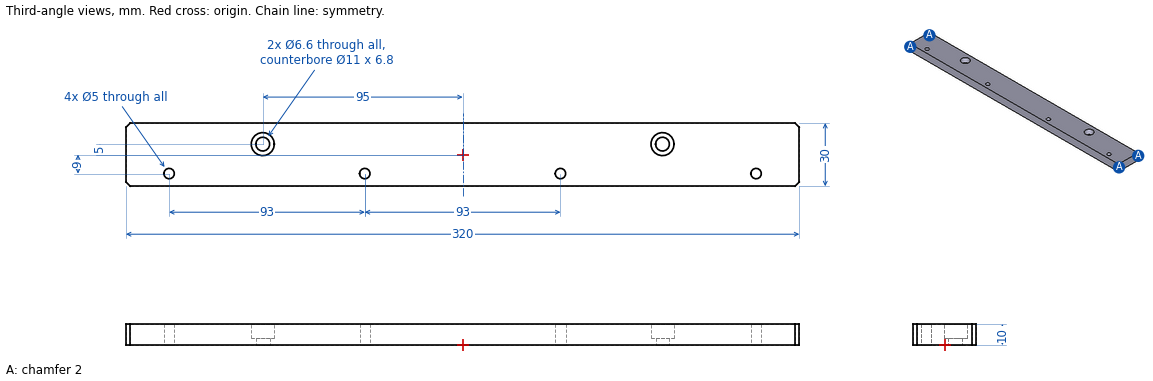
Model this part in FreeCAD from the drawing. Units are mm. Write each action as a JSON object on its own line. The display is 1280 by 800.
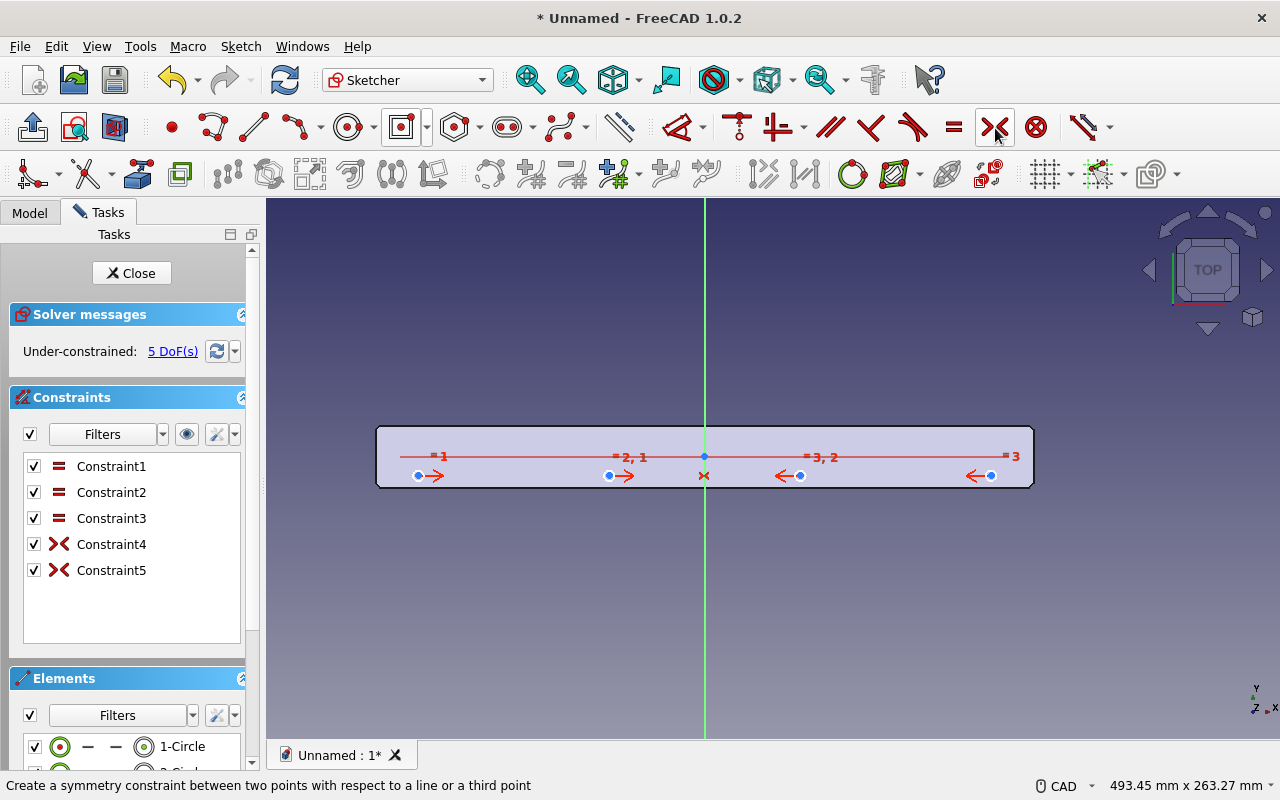
{"action": "left_click", "coordinate": [676, 128]}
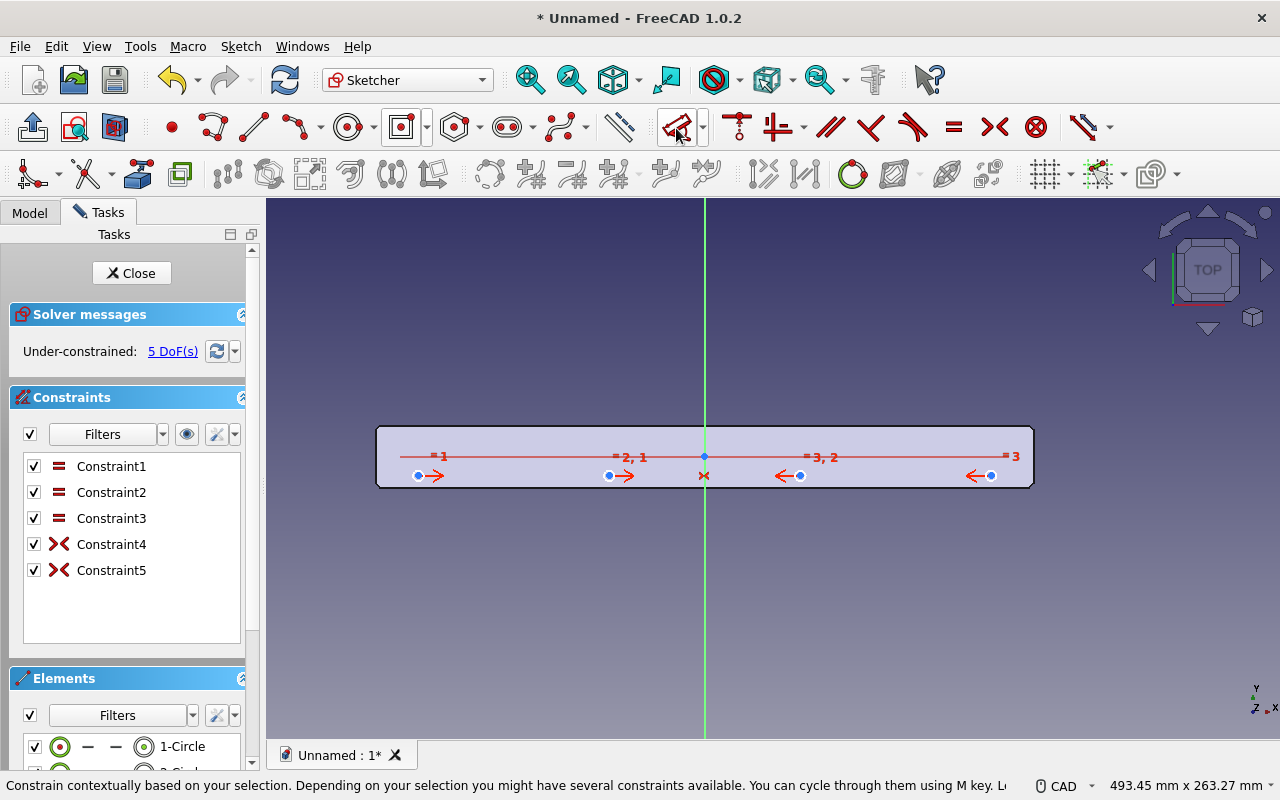
{"action": "scroll", "coordinate": [415, 480], "scroll_direction": "up", "scroll_amount": 7}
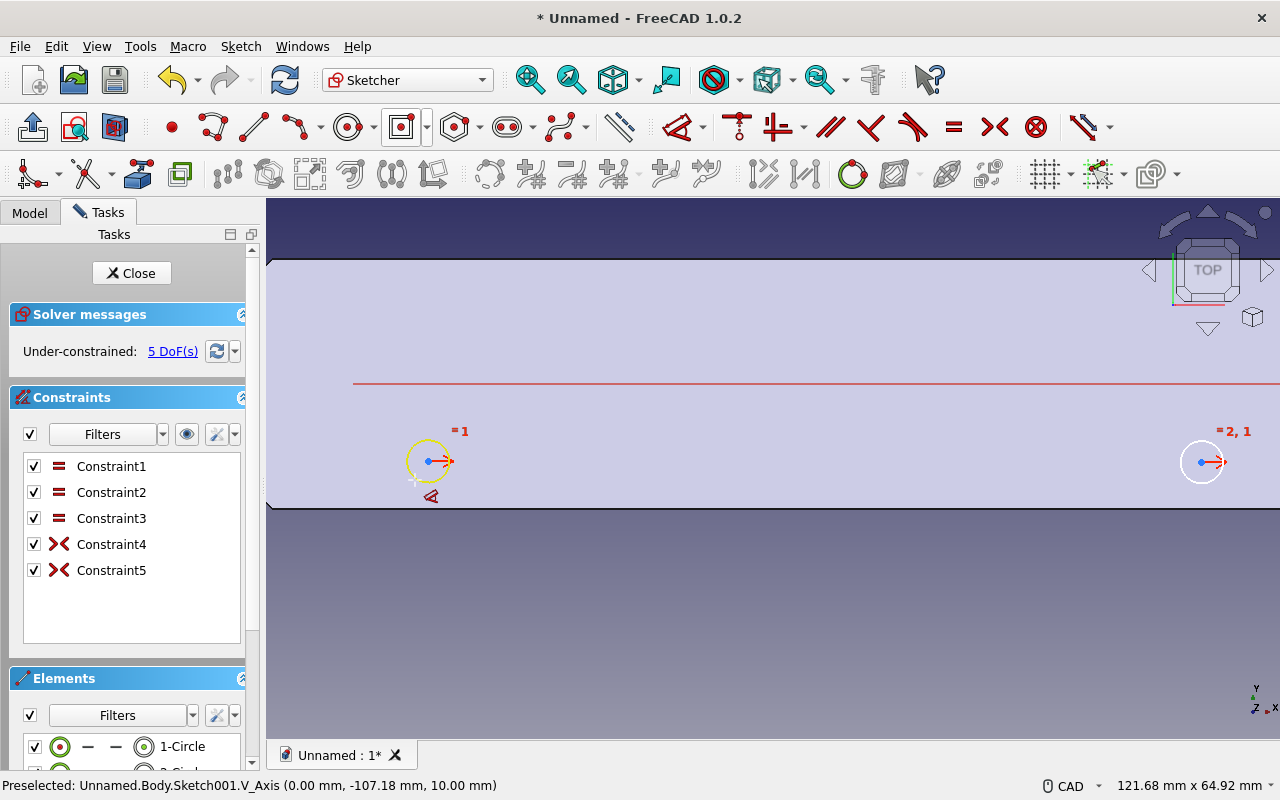
{"action": "left_click", "coordinate": [413, 476]}
{"action": "left_click", "coordinate": [390, 498]}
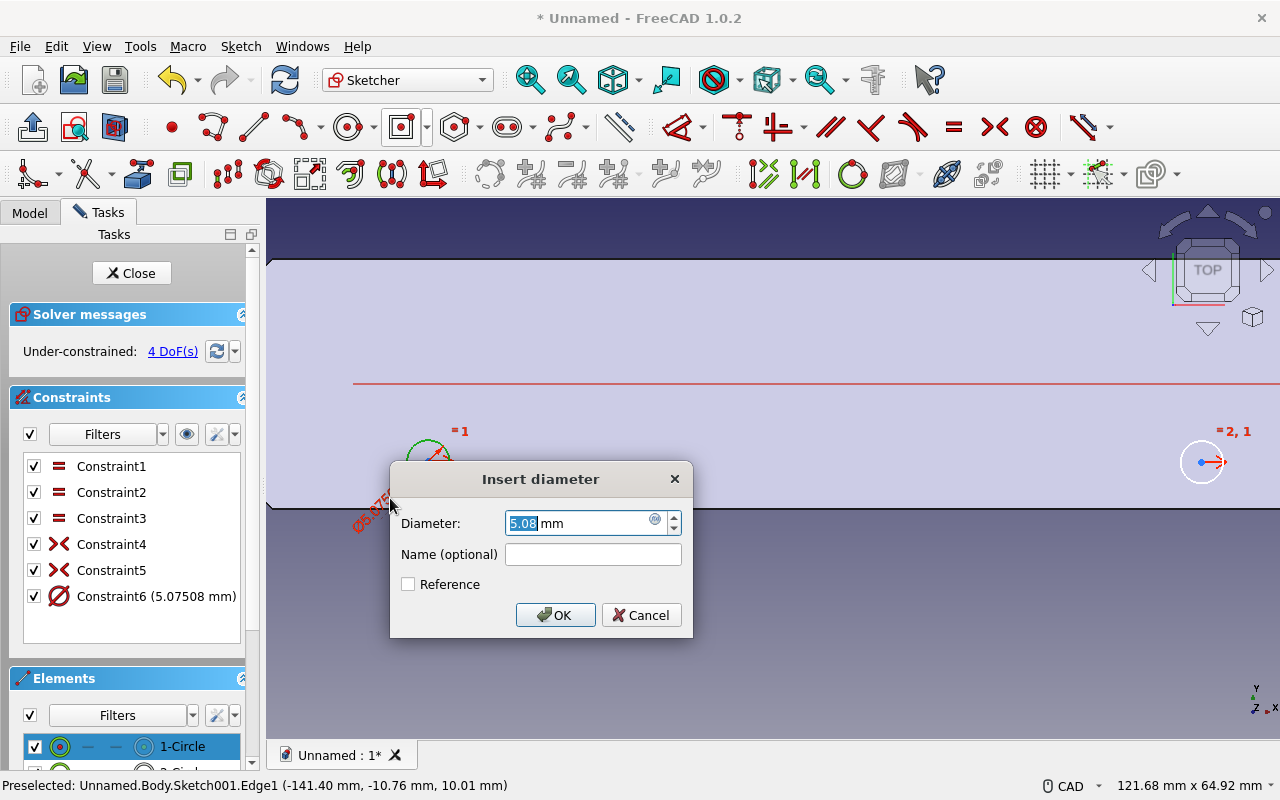
{"action": "type", "text": "5"}
{"action": "key", "text": "Return"}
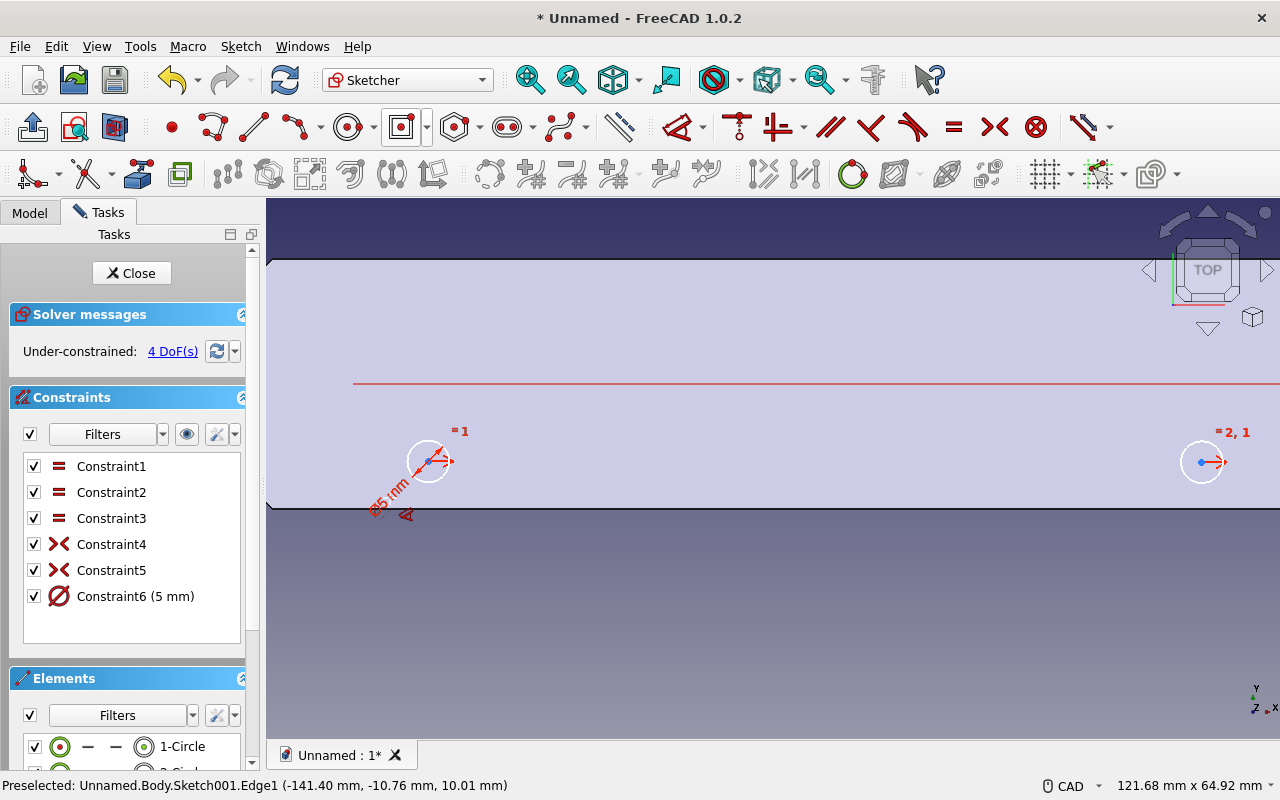
{"action": "left_click", "coordinate": [428, 461]}
{"action": "left_click", "coordinate": [394, 423]}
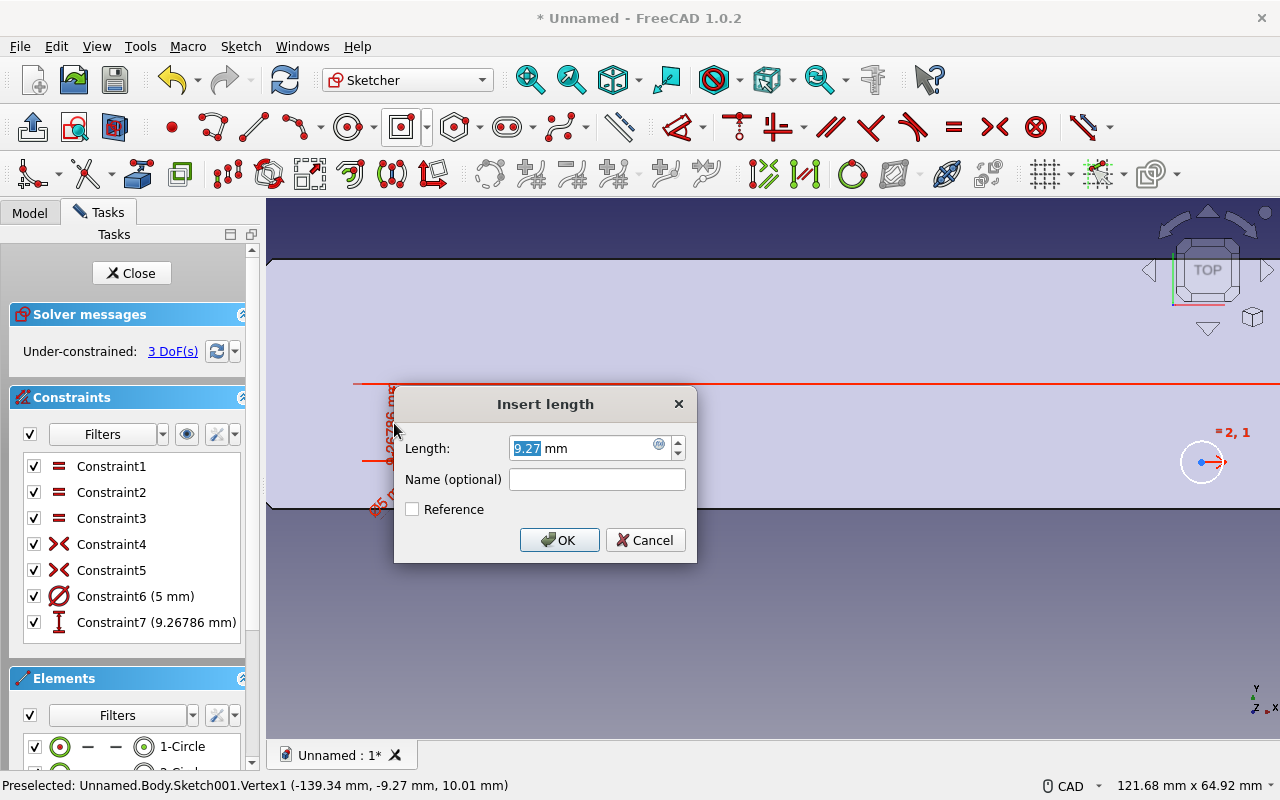
{"action": "type", "text": "9"}
{"action": "key", "text": "Return"}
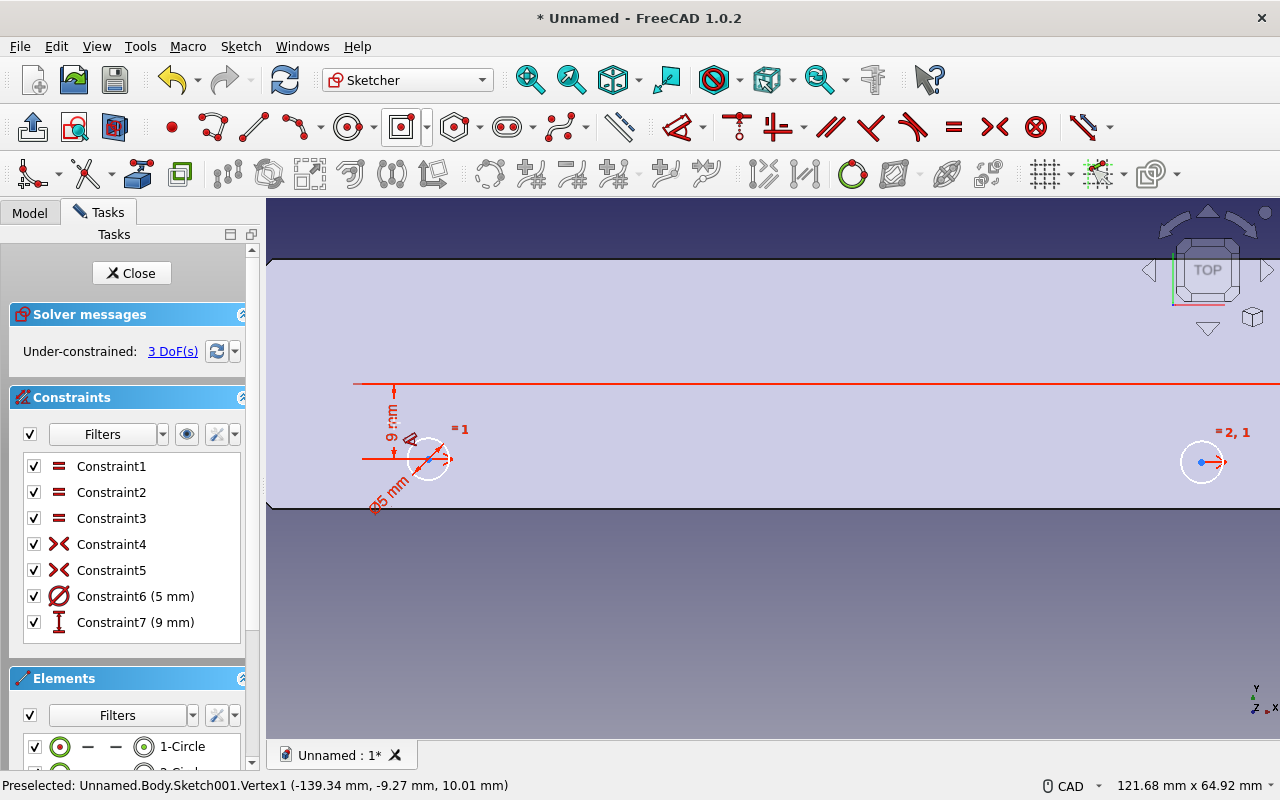
{"action": "scroll", "coordinate": [415, 480], "scroll_direction": "down", "scroll_amount": 7}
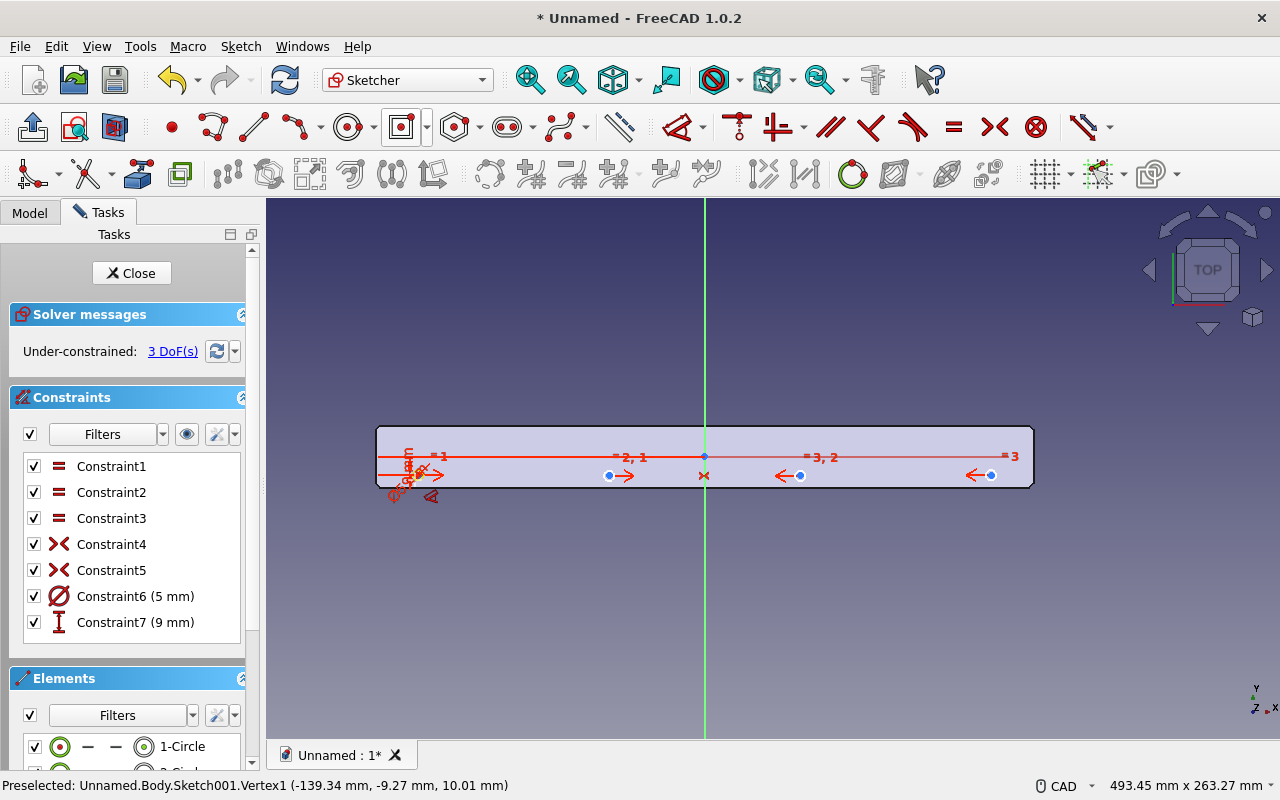
{"action": "scroll", "coordinate": [609, 476], "scroll_direction": "up", "scroll_amount": 4}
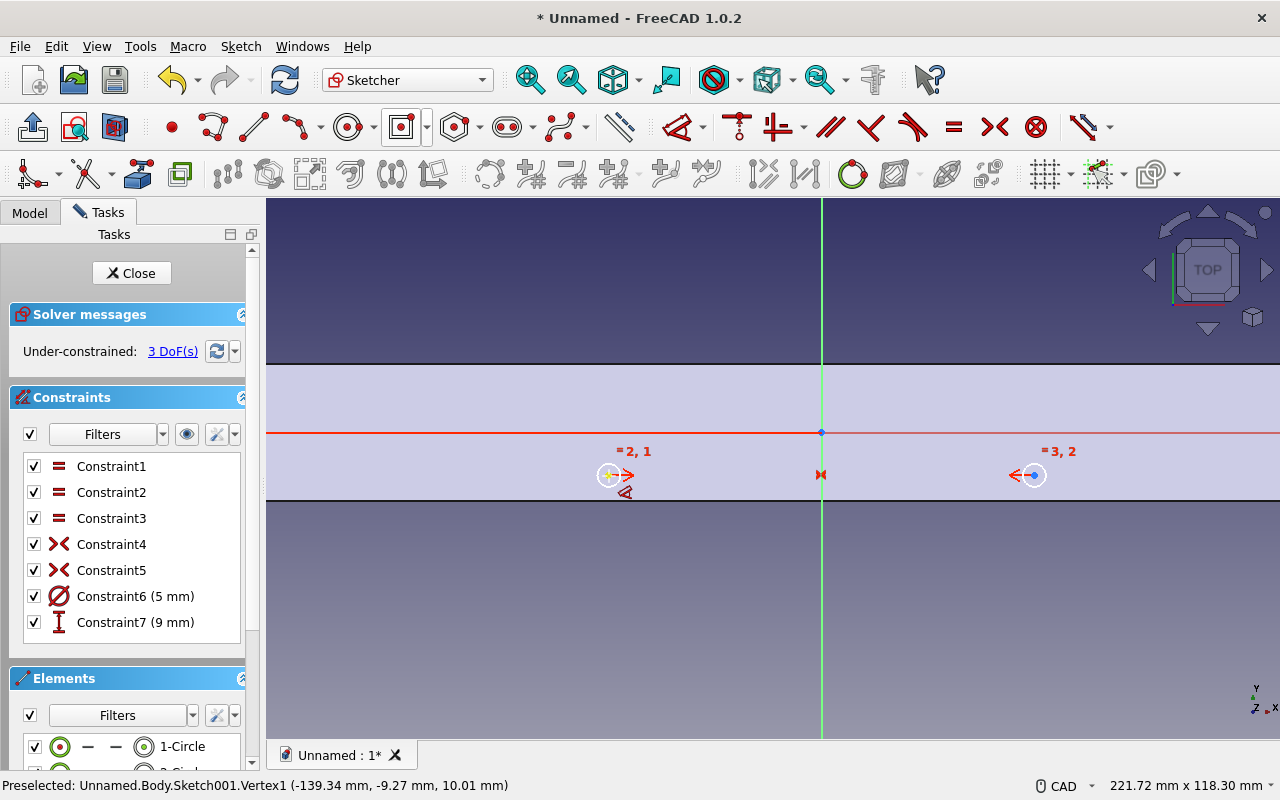
{"action": "left_click", "coordinate": [609, 475]}
{"action": "left_click", "coordinate": [575, 454]}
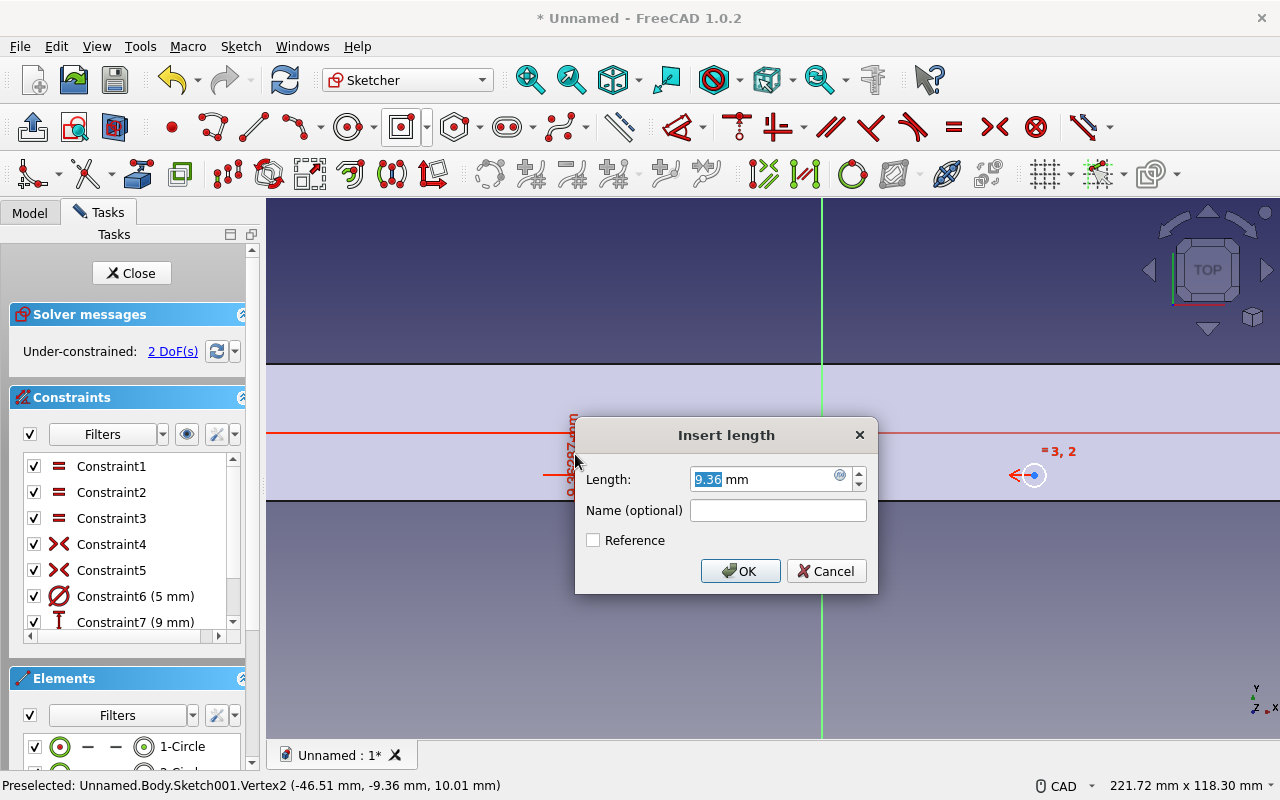
{"action": "type", "text": "9"}
{"action": "key", "text": "Return"}